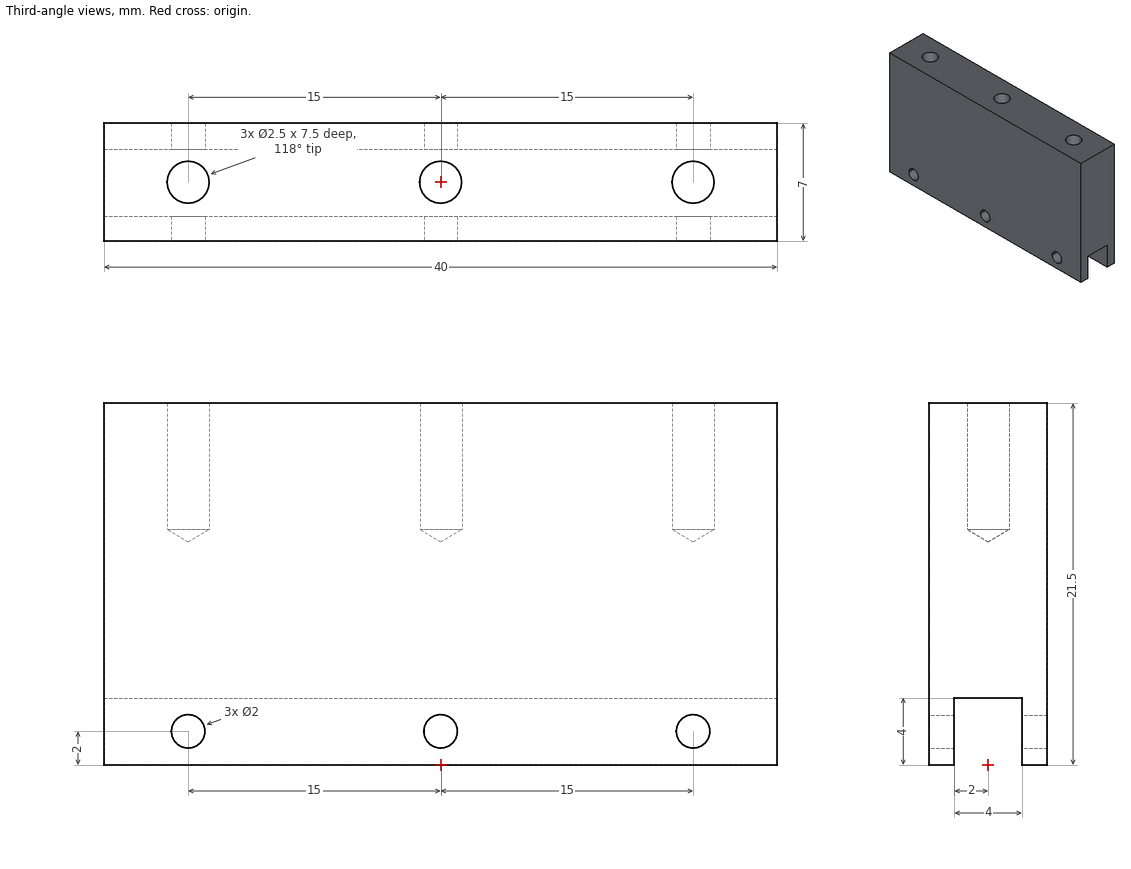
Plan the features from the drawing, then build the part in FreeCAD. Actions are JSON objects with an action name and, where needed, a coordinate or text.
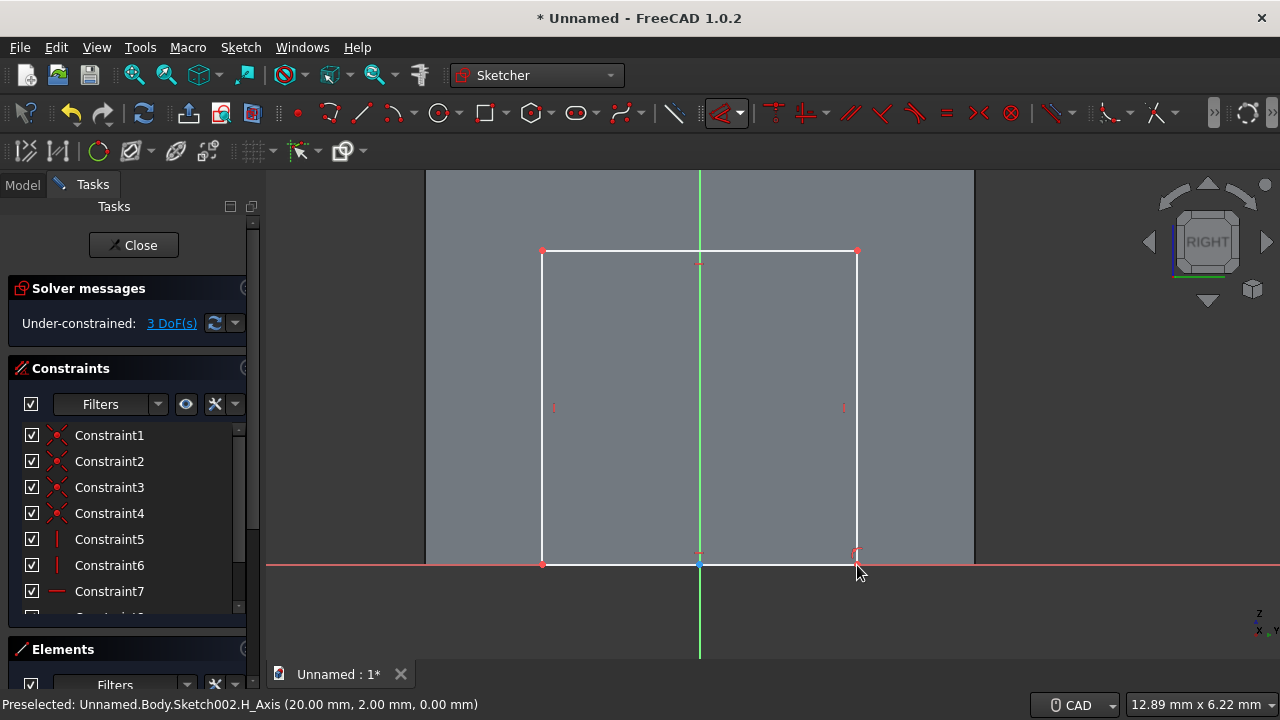
{"action": "left_click", "coordinate": [542, 345]}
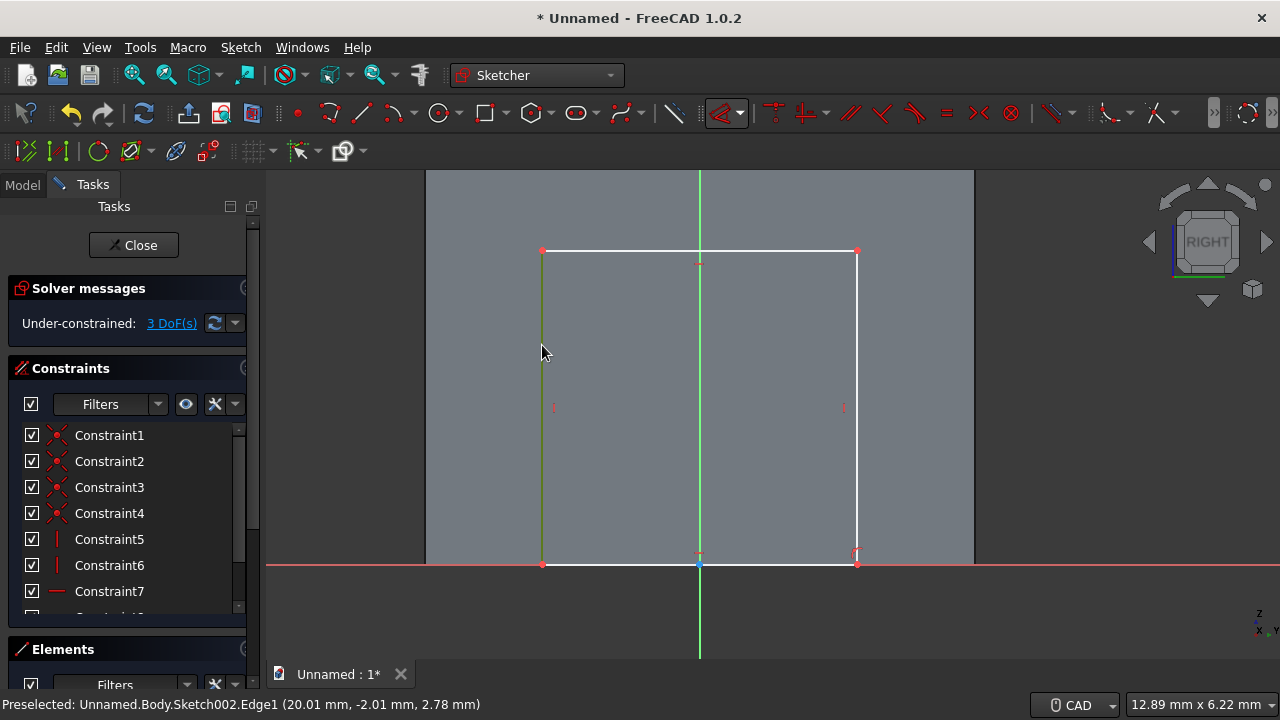
{"action": "key", "text": "i"}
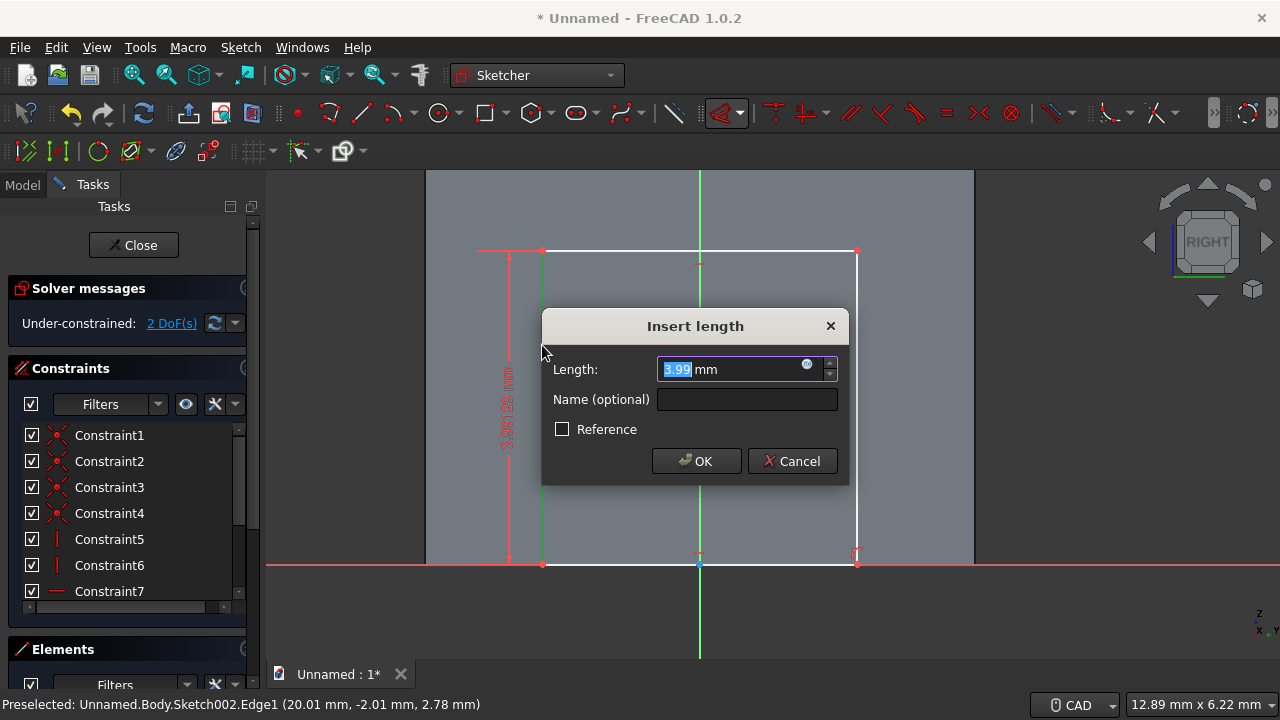
{"action": "type", "text": "4"}
{"action": "key", "text": "Return"}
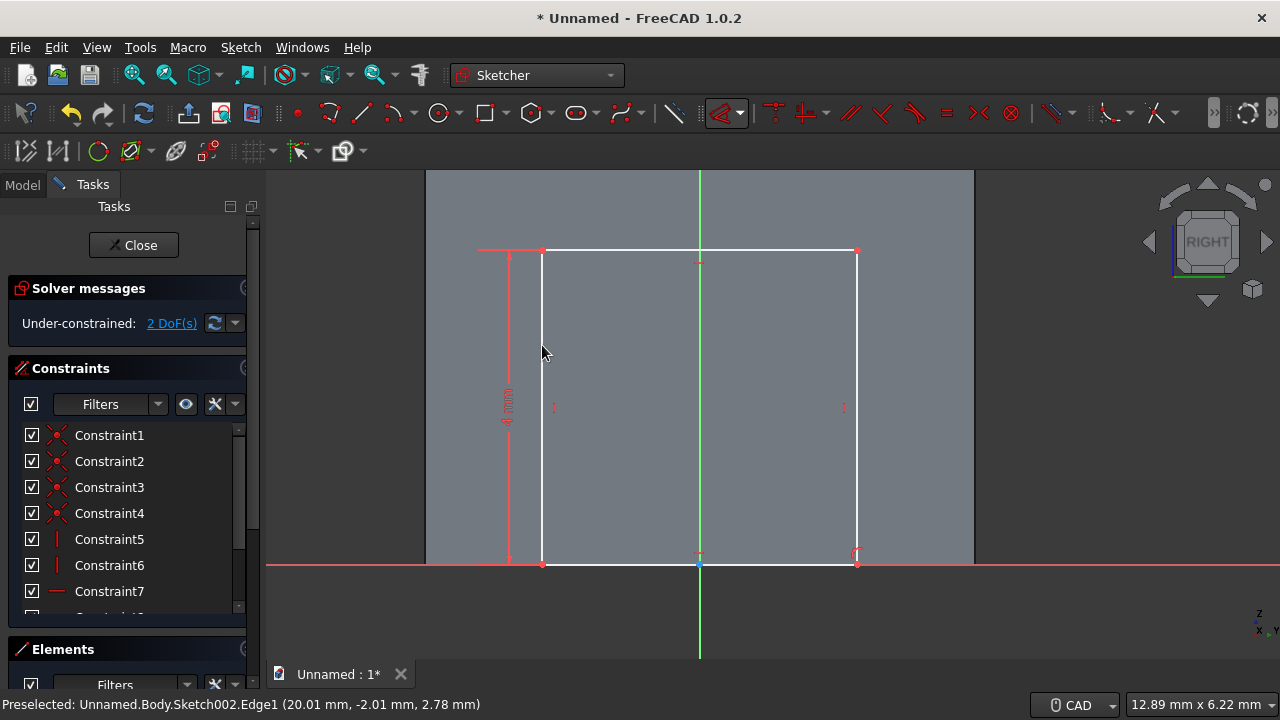
{"action": "left_click", "coordinate": [637, 565]}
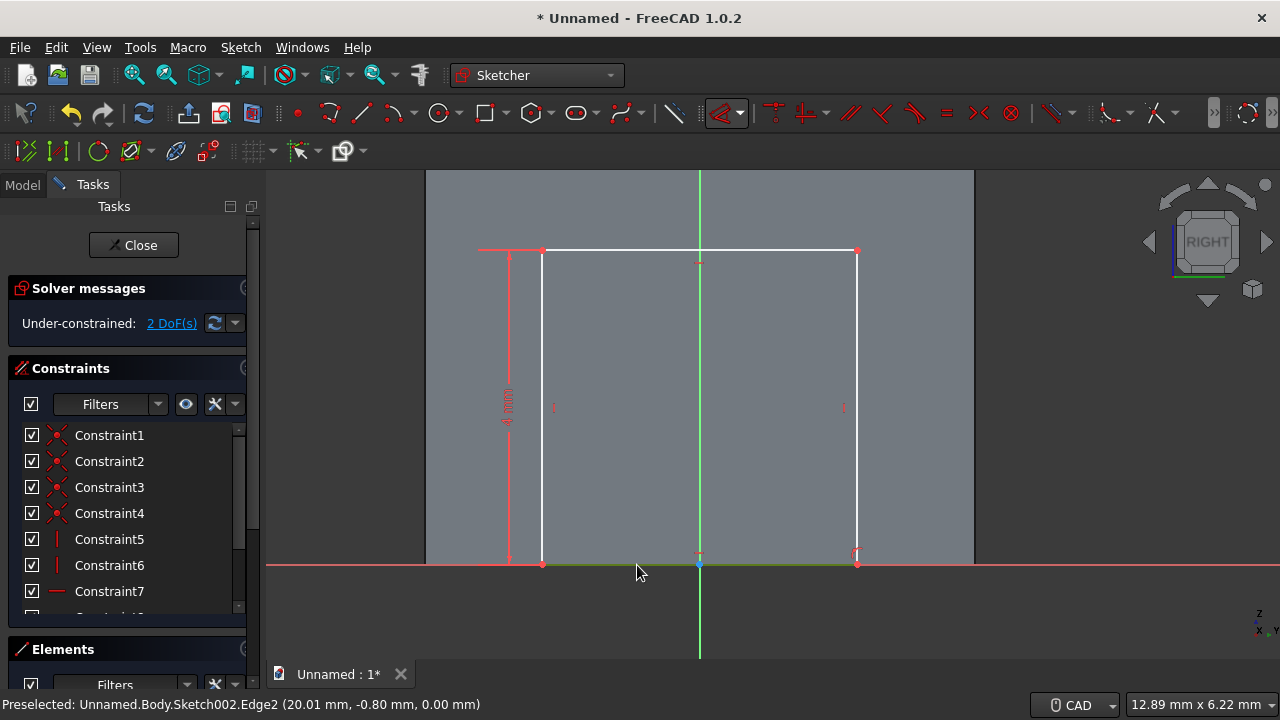
{"action": "left_click", "coordinate": [742, 114]}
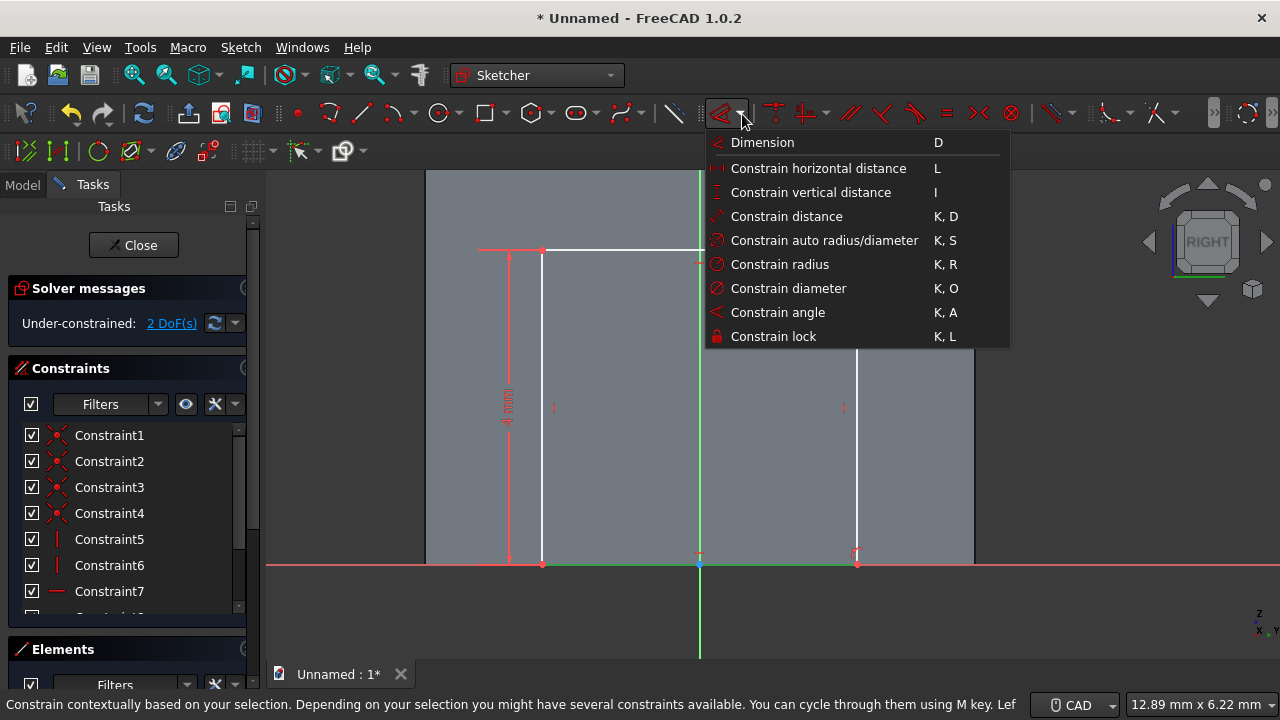
{"action": "left_click", "coordinate": [858, 168]}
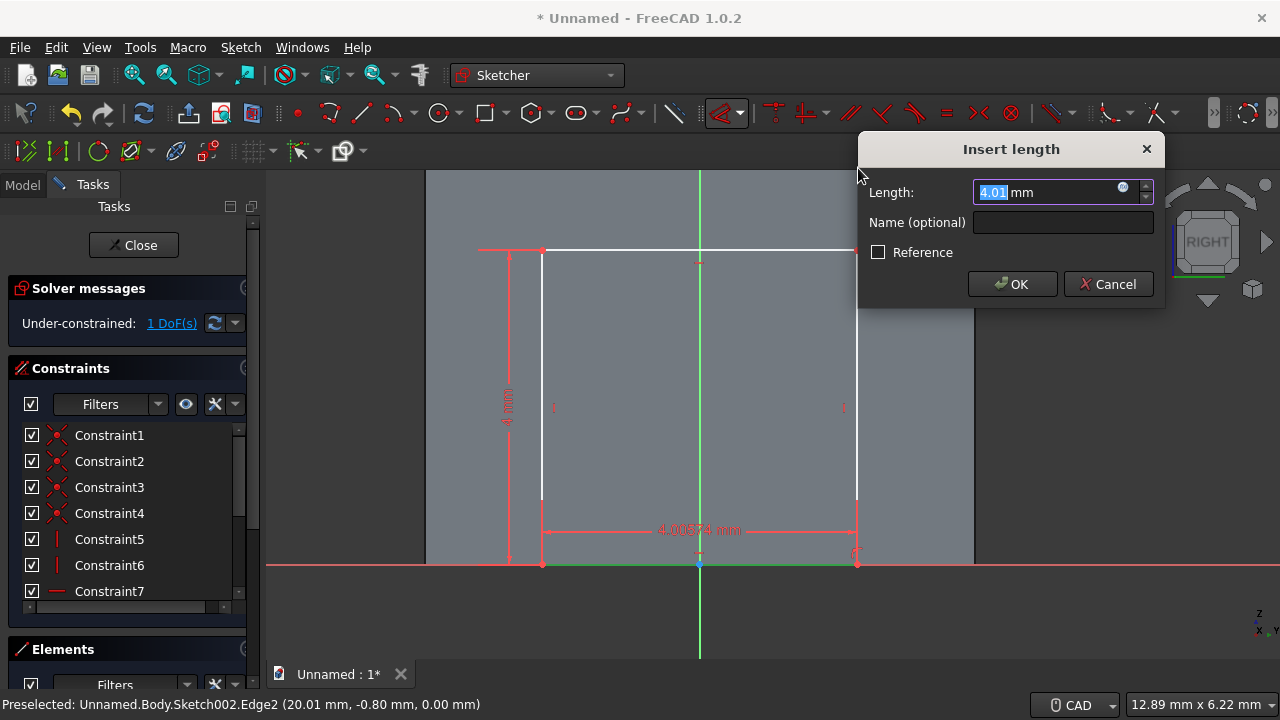
{"action": "type", "text": "4"}
{"action": "key", "text": "Return"}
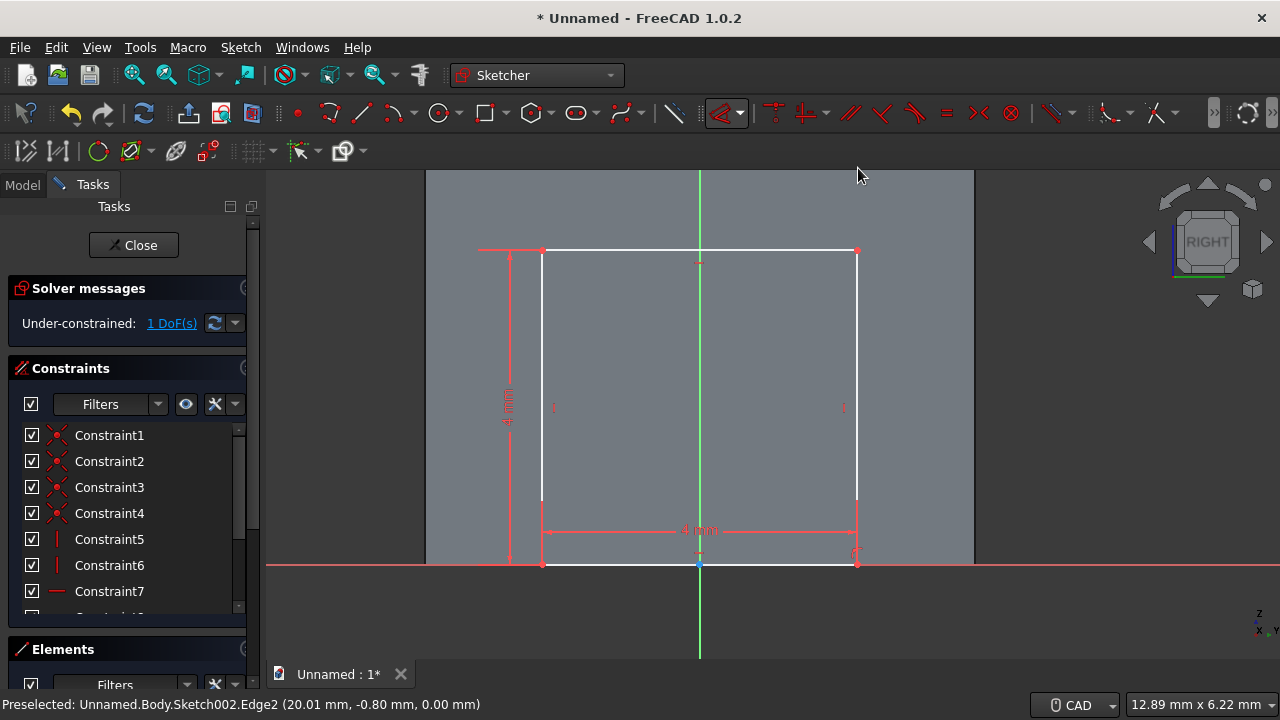
{"action": "left_click", "coordinate": [542, 250]}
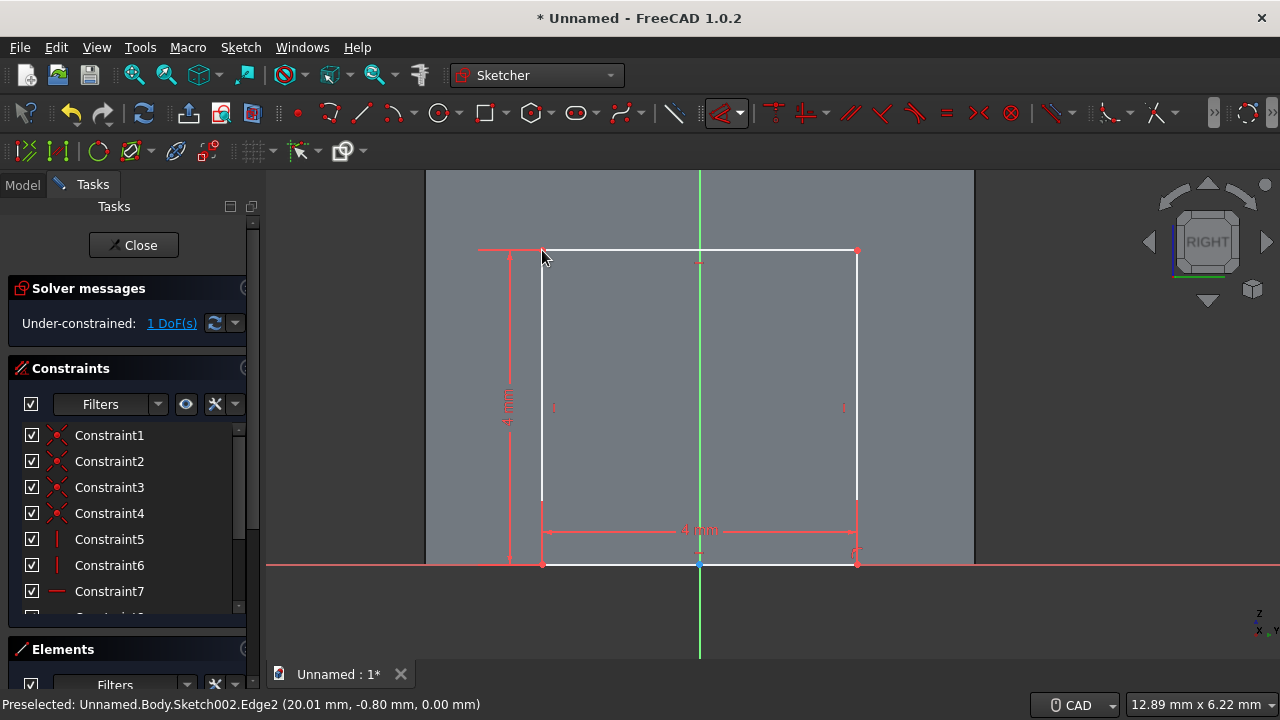
{"action": "left_click", "coordinate": [742, 114]}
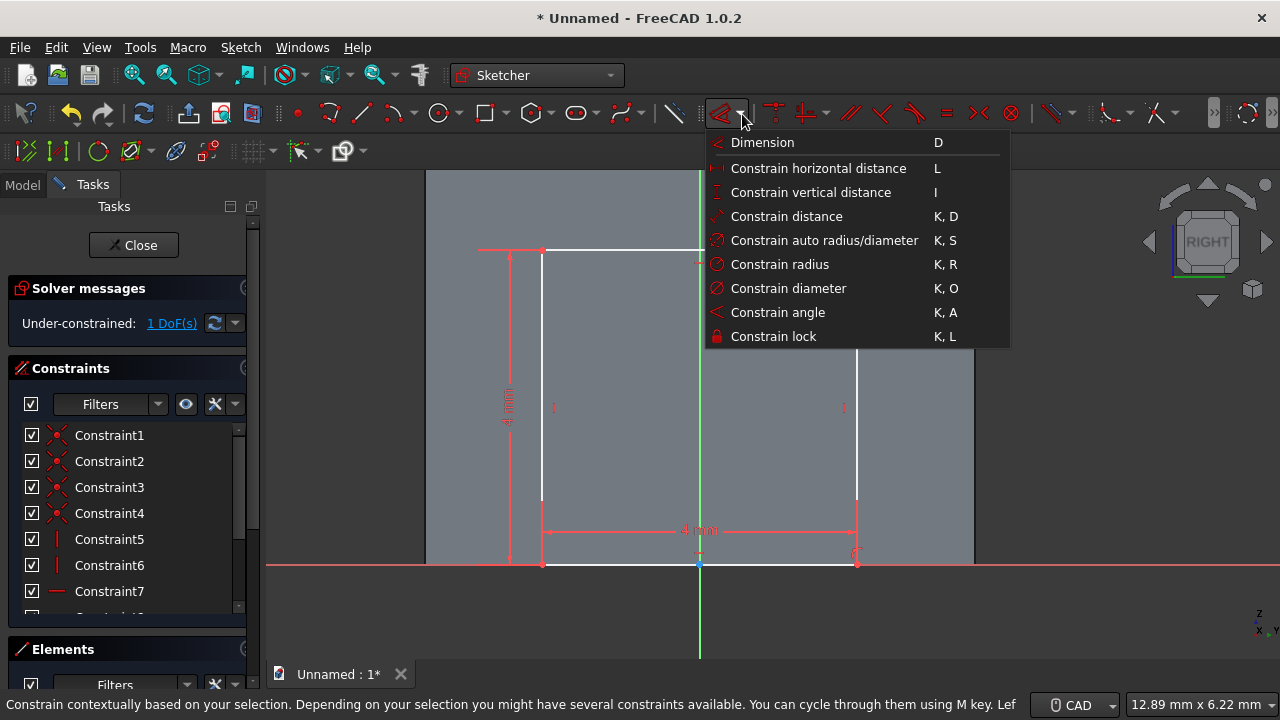
{"action": "left_click", "coordinate": [858, 168]}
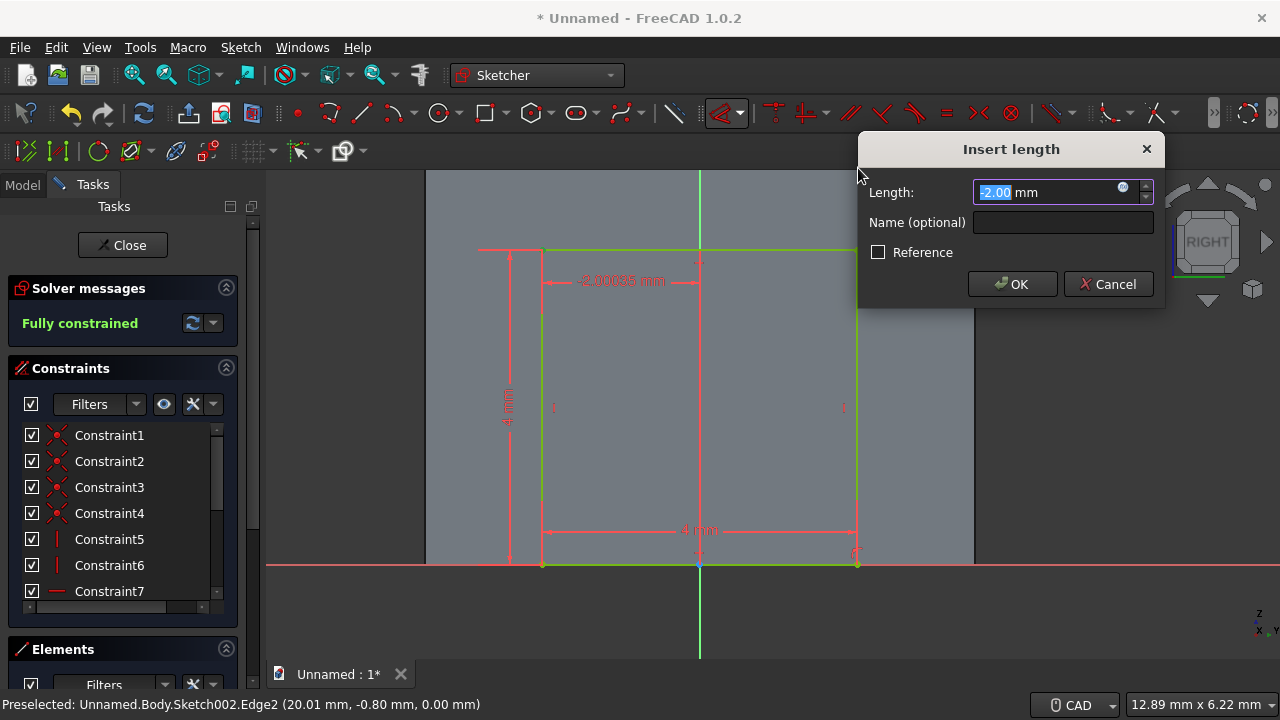
{"action": "type", "text": "-2"}
{"action": "key", "text": "Return"}